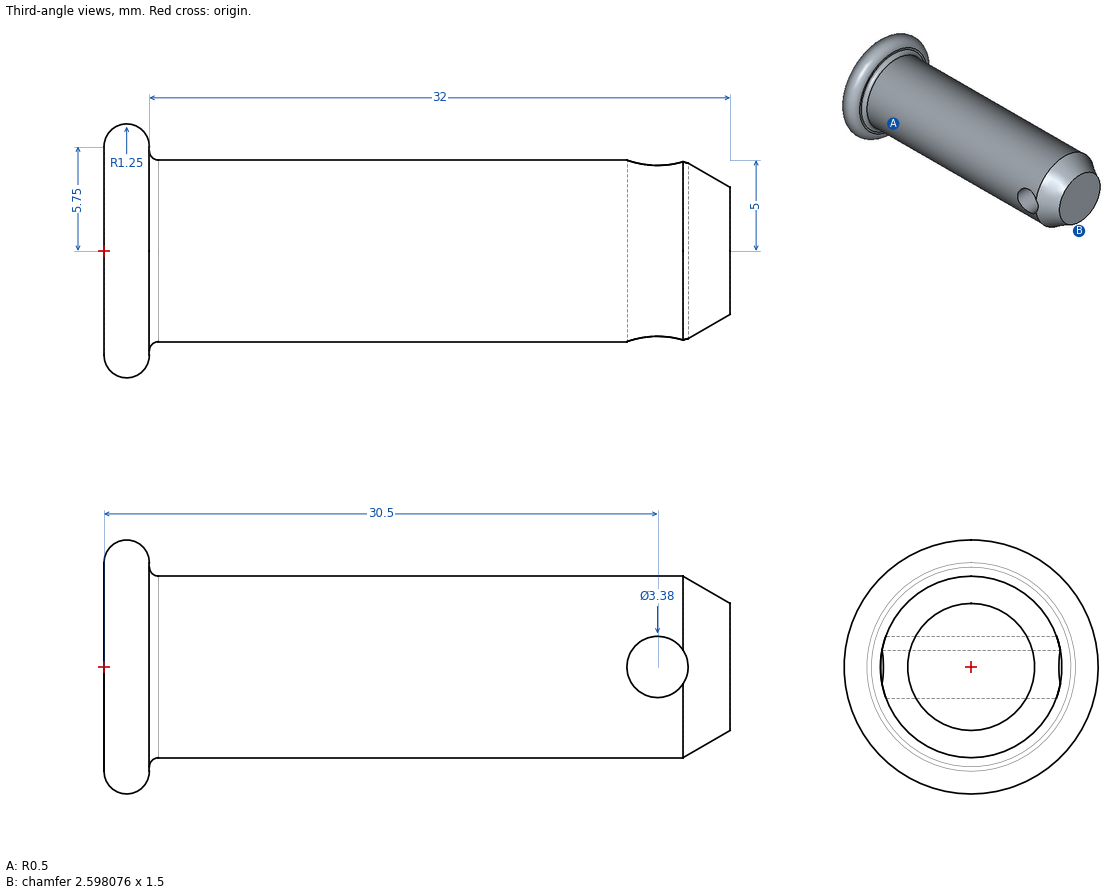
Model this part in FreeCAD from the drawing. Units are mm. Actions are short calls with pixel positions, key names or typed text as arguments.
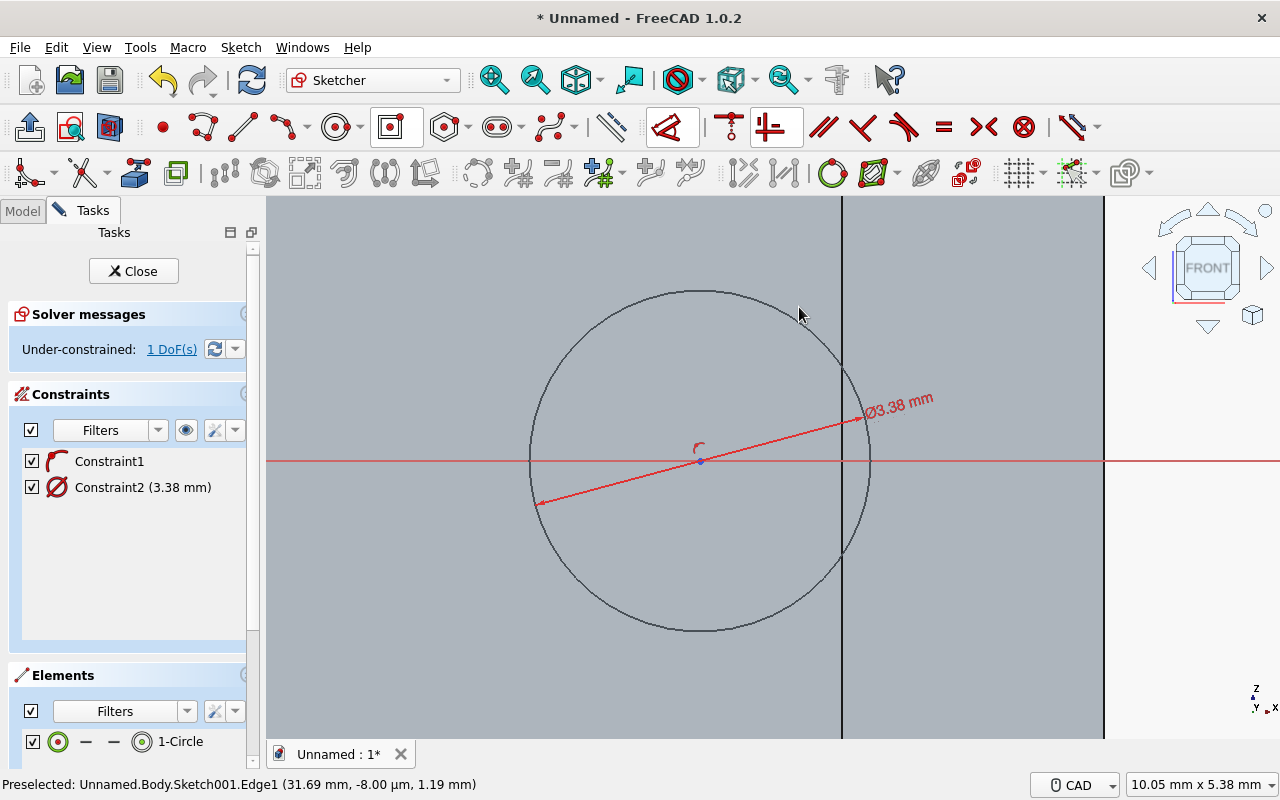
click(700, 461)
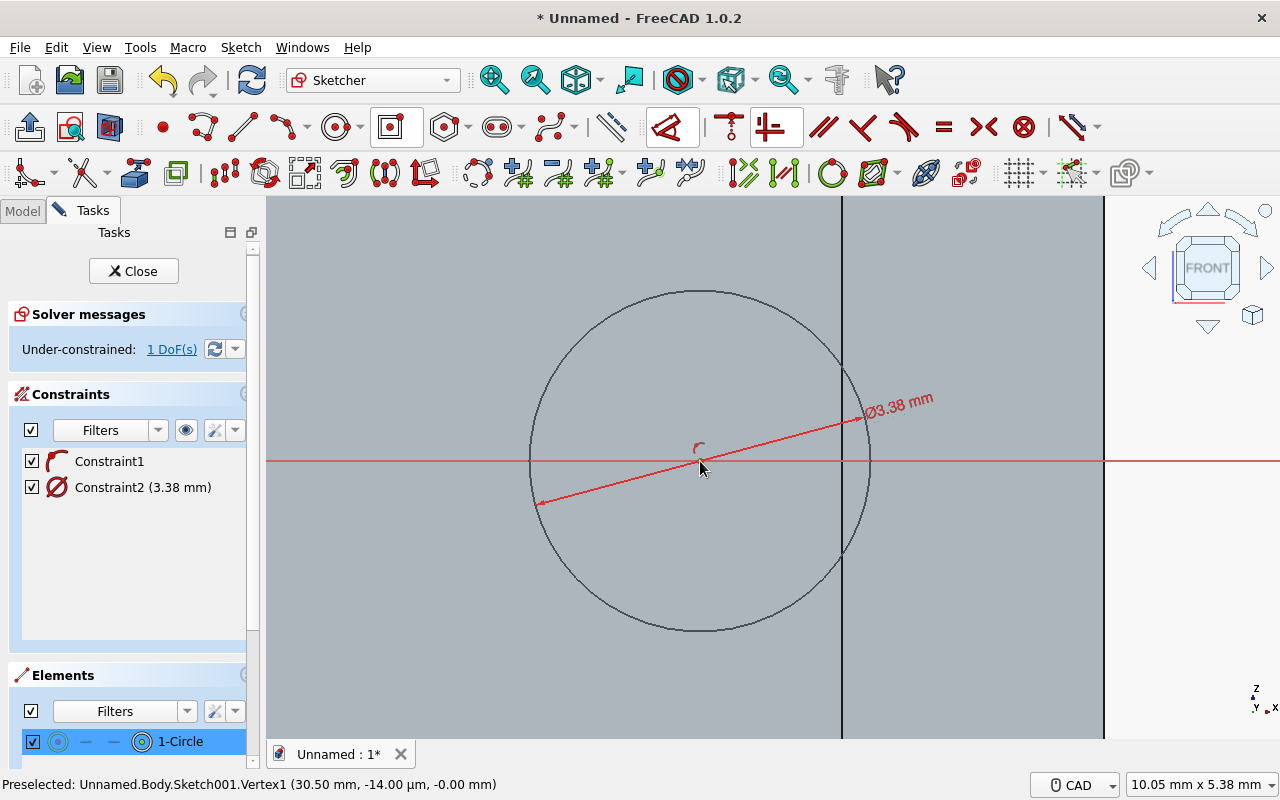
key(l)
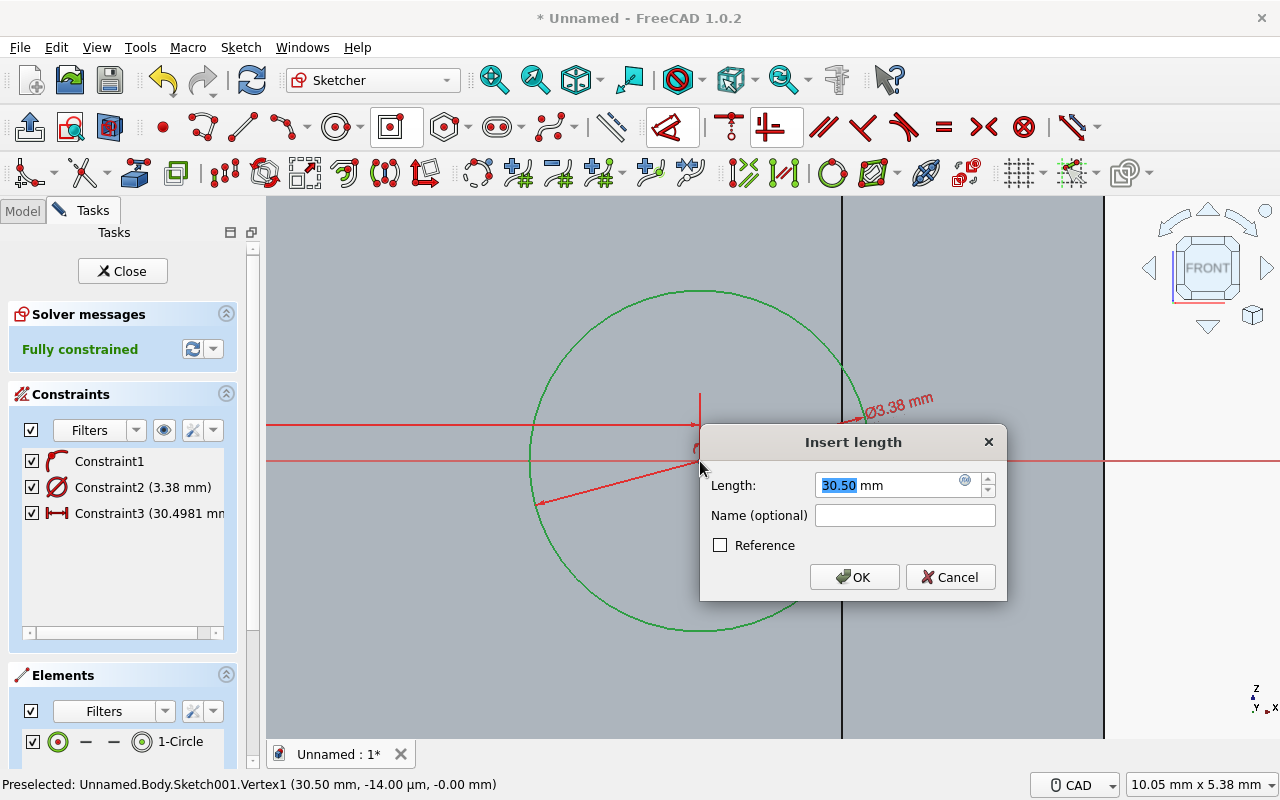
text(30.5)
key(Return)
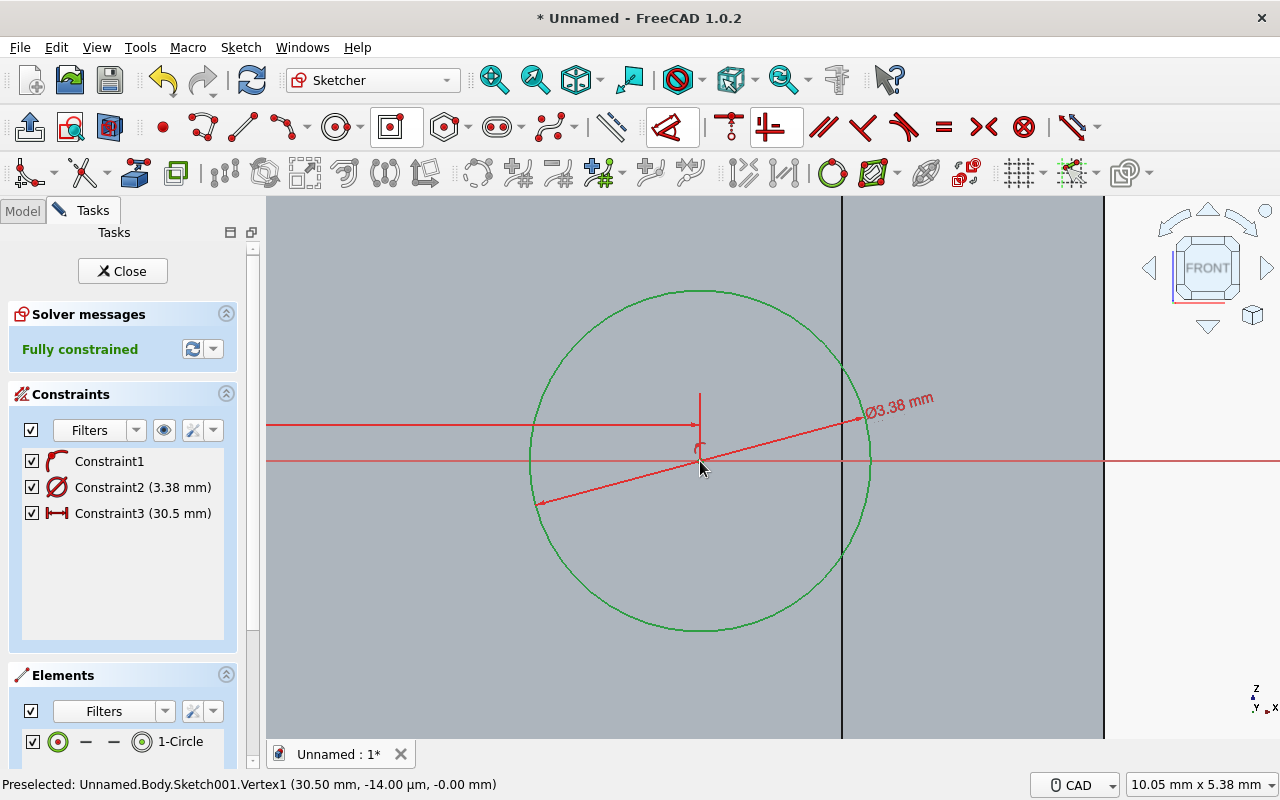
click(123, 271)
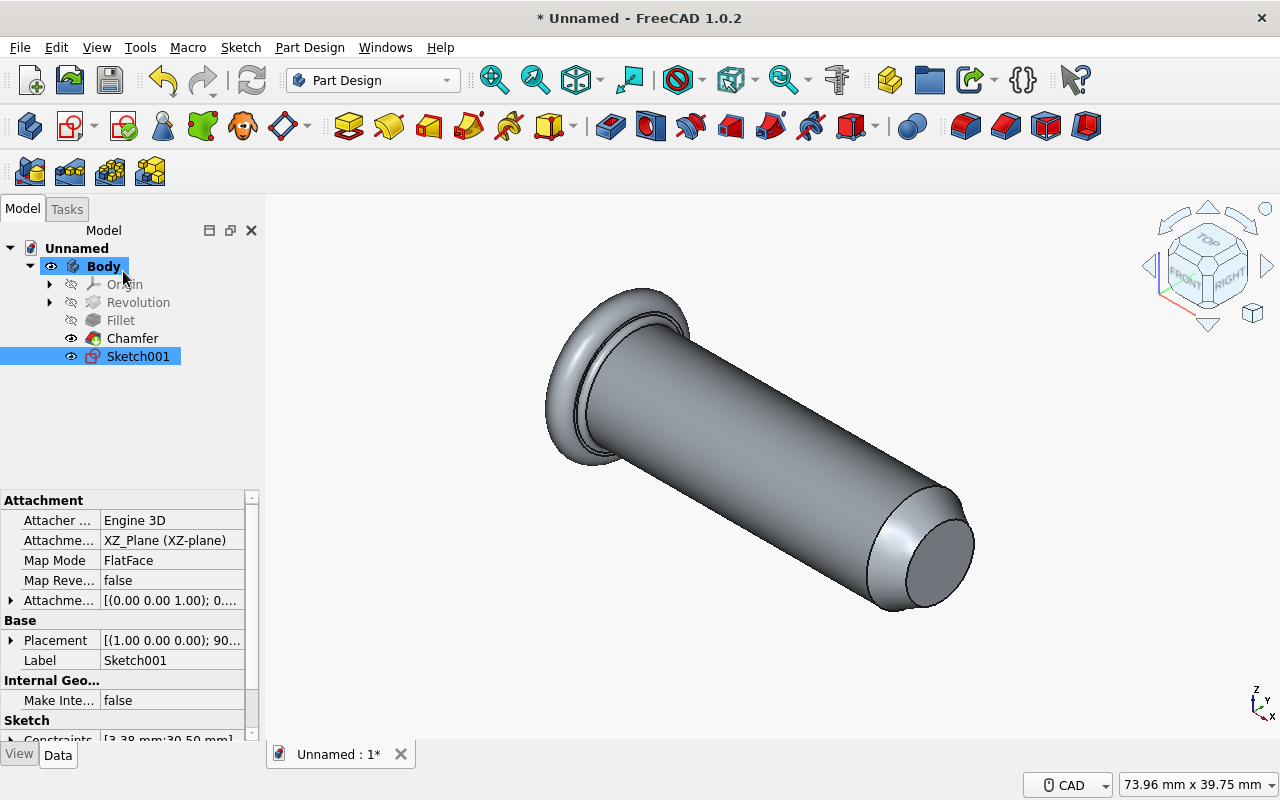
click(612, 126)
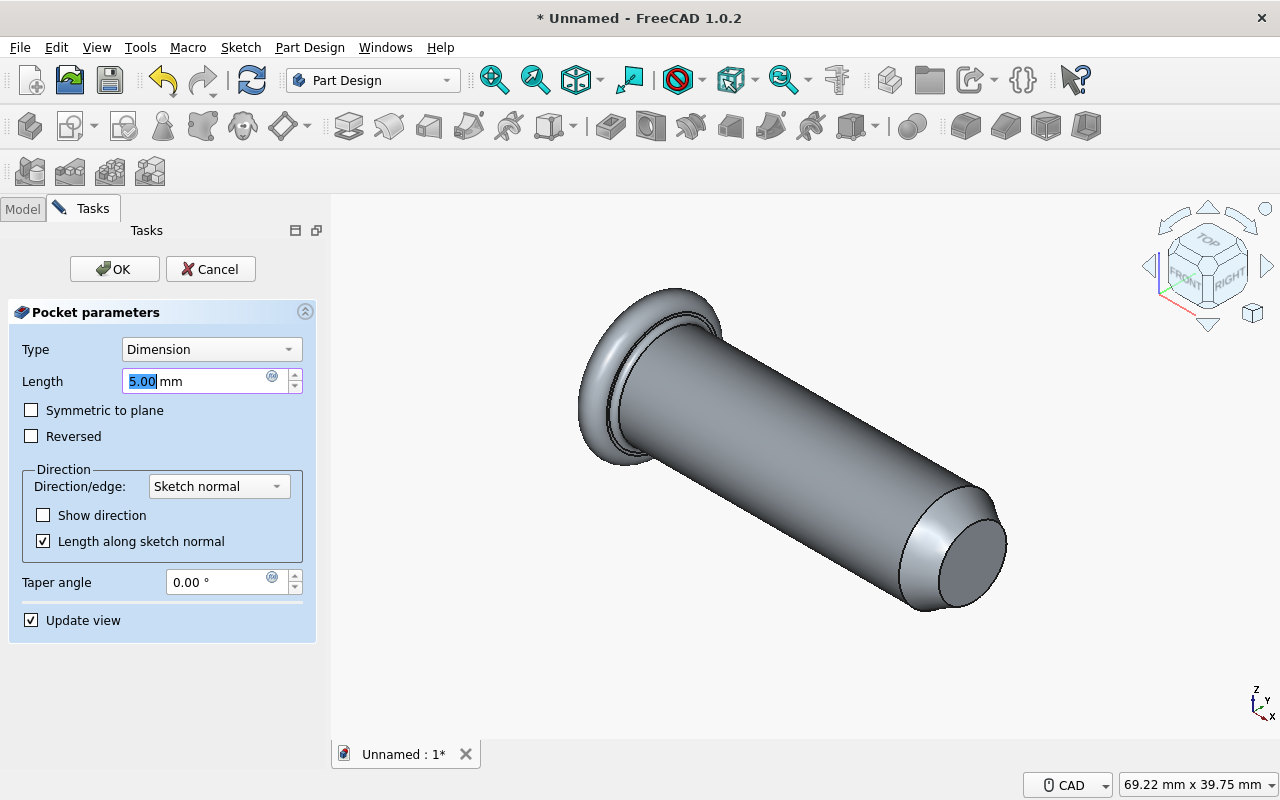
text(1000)
key(Tab)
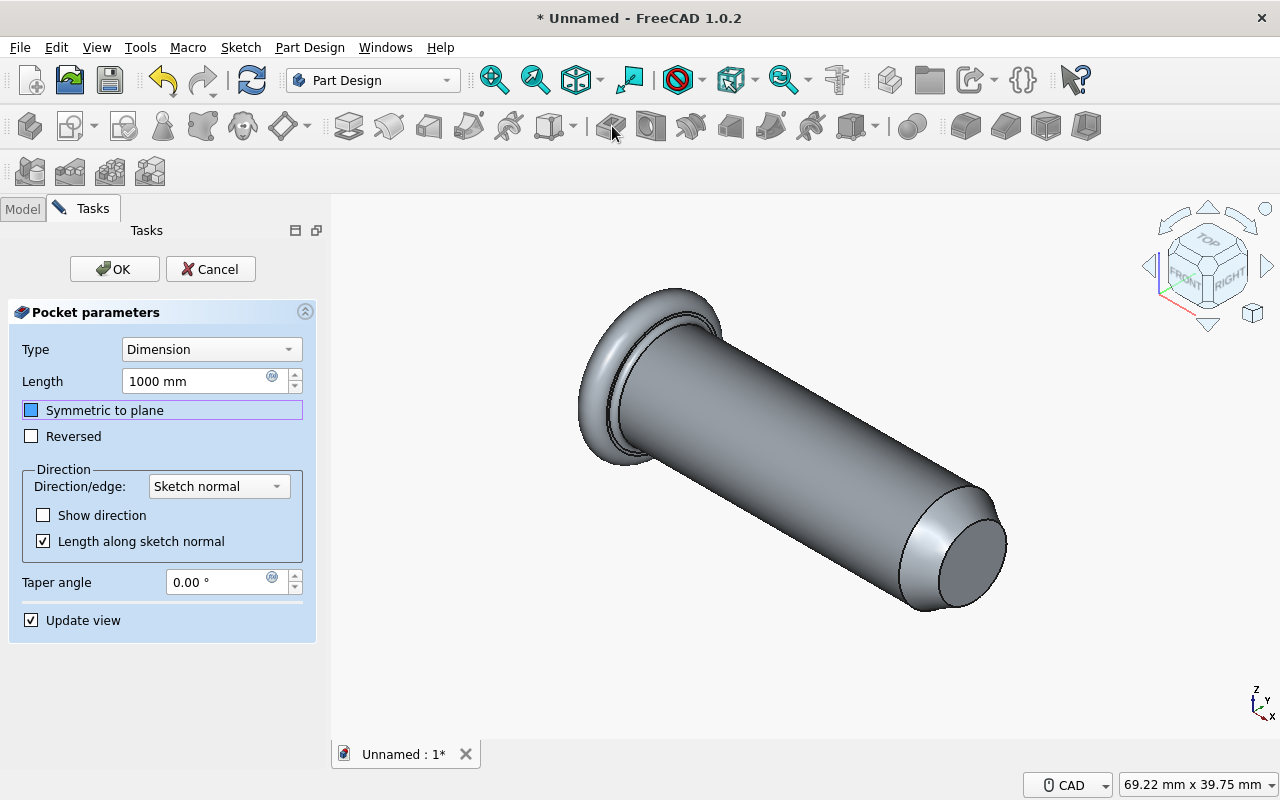
click(30, 410)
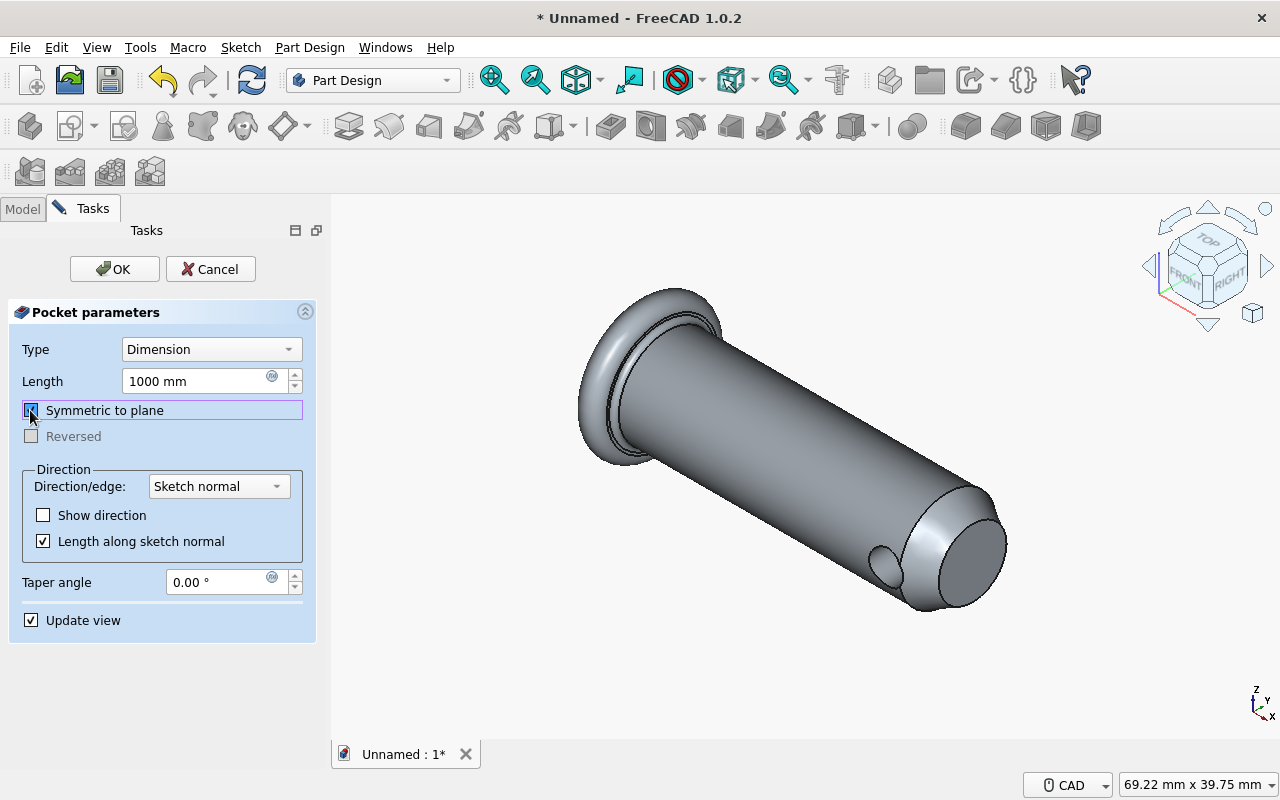
click(115, 269)